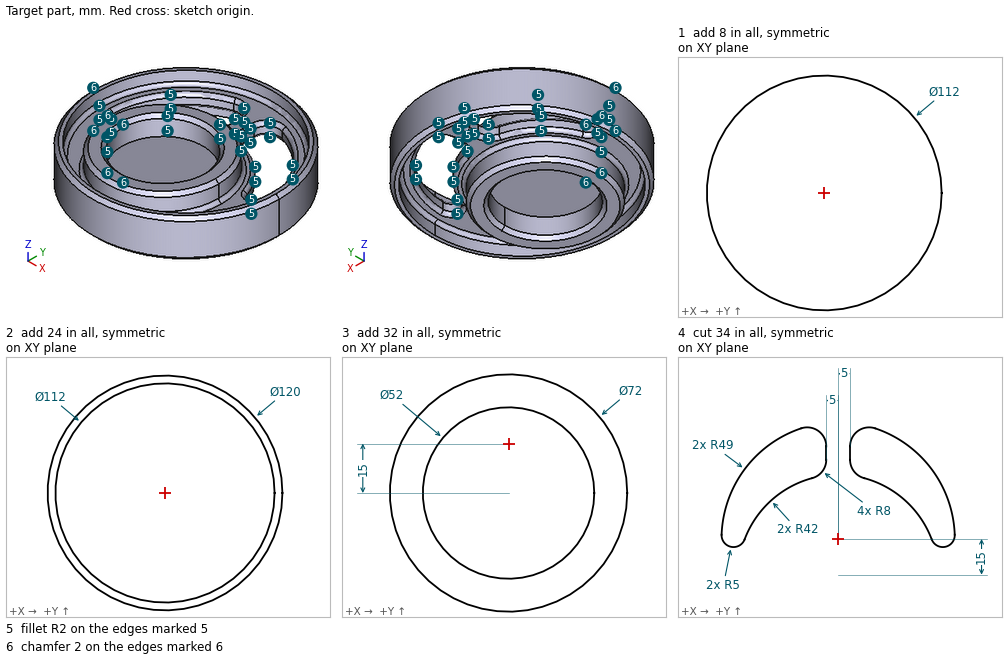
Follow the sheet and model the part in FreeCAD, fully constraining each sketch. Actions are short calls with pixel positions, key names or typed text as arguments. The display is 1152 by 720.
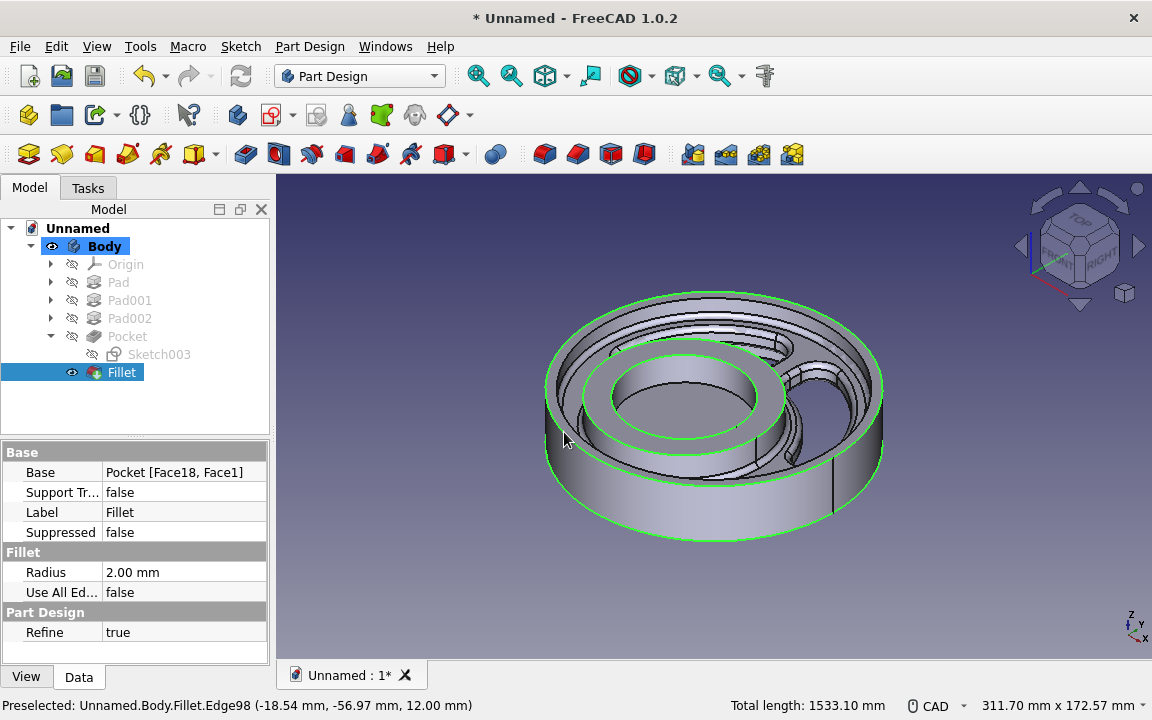
click(578, 154)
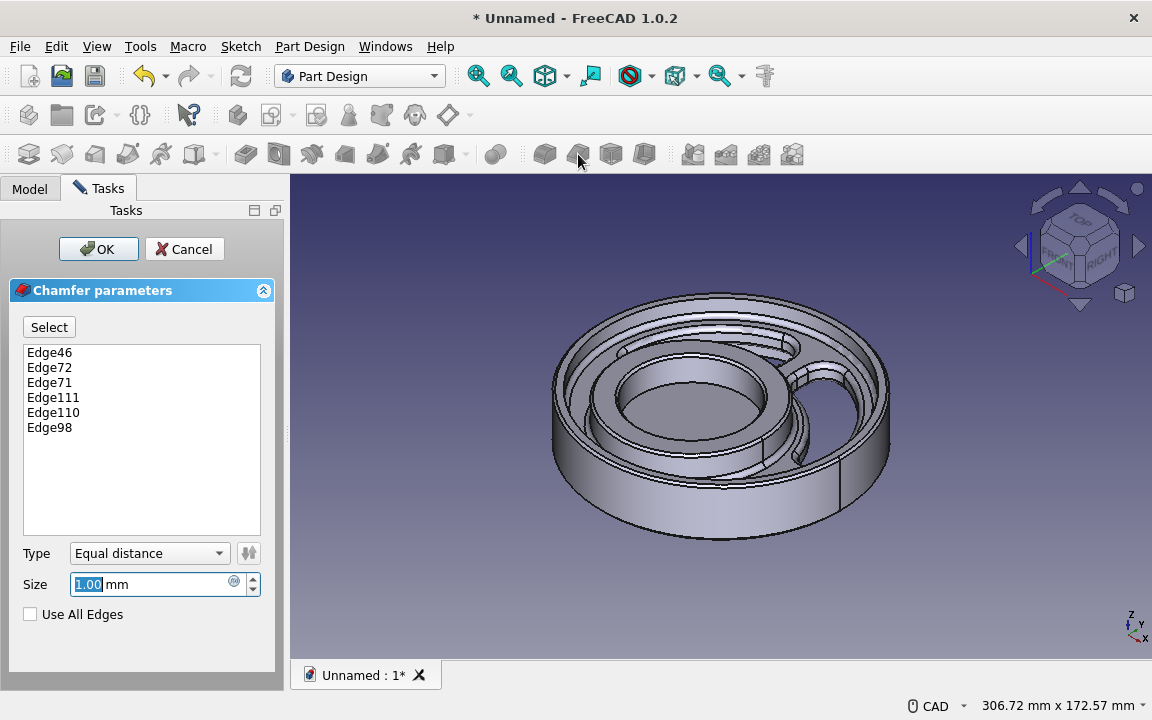
text(2)
key(Tab)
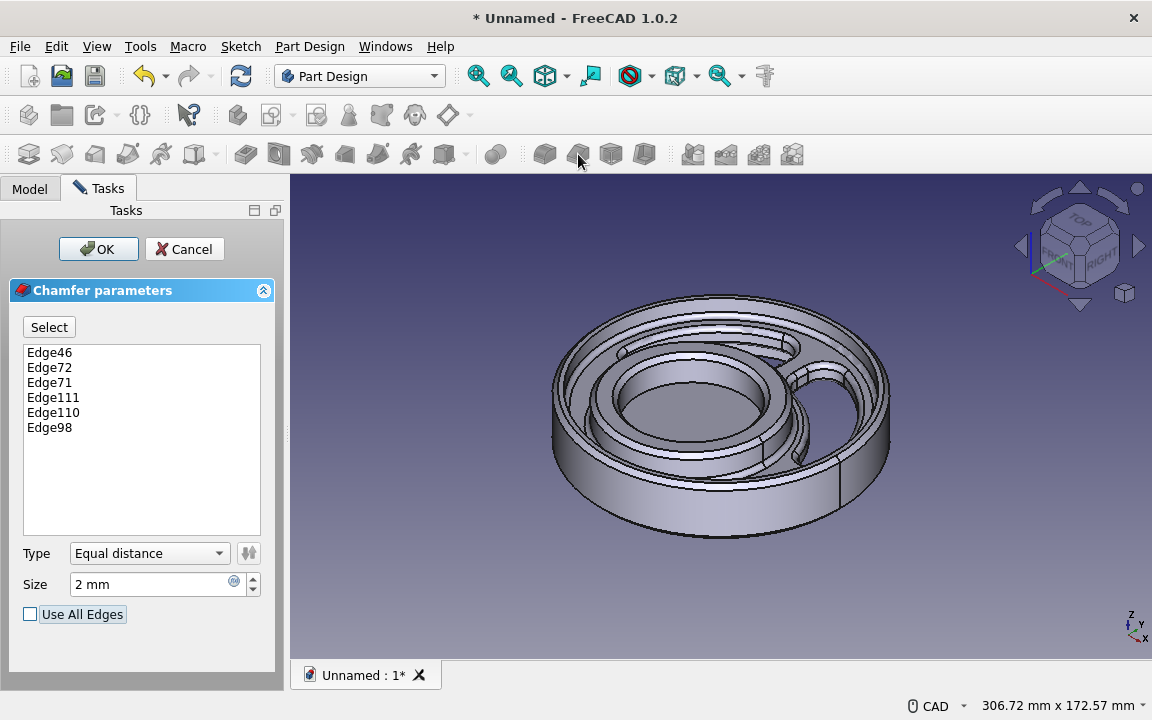
click(99, 249)